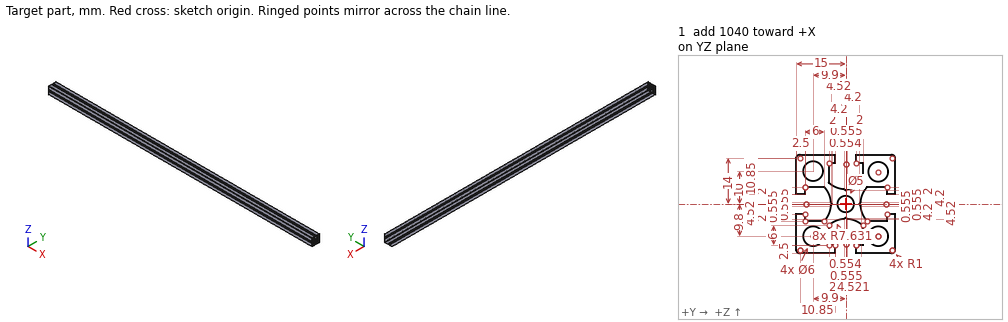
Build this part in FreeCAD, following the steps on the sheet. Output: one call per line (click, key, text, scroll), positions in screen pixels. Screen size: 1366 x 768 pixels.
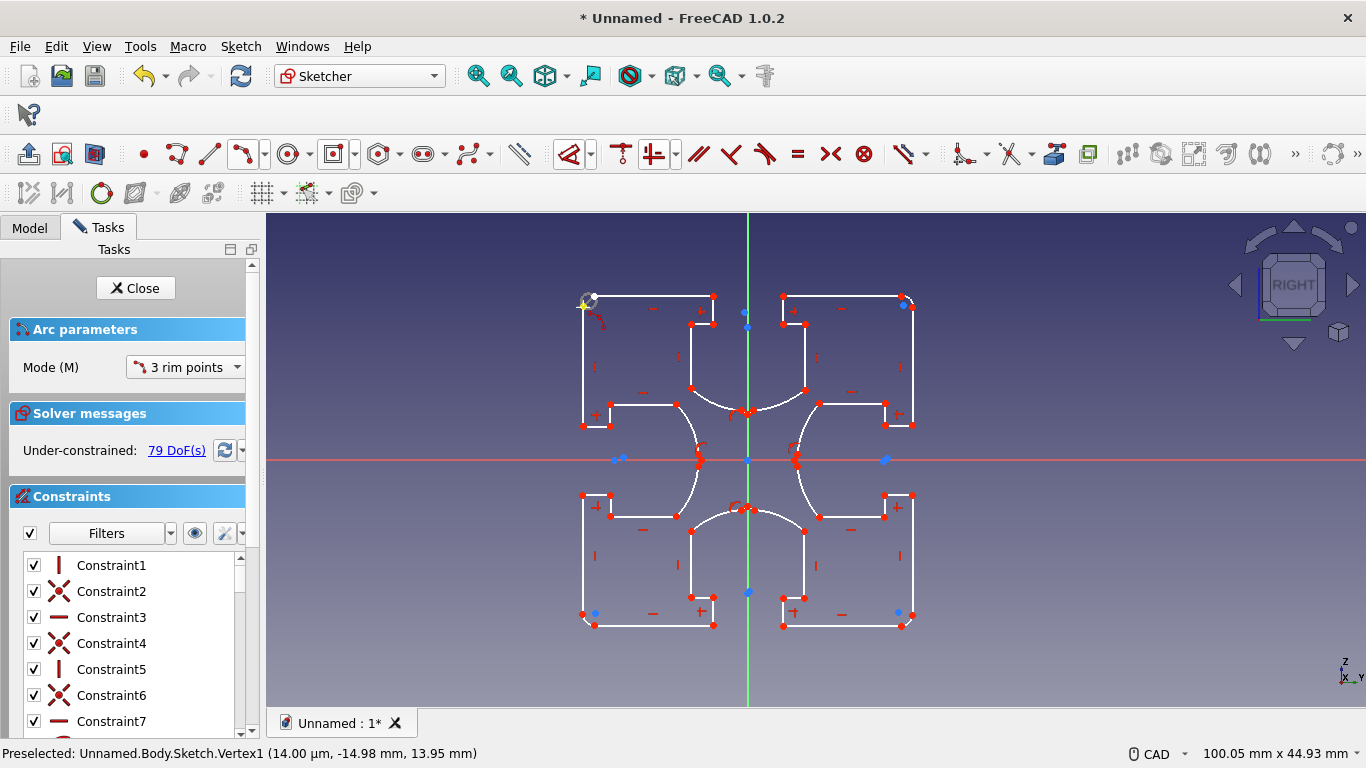
scroll(586, 298, up, 8)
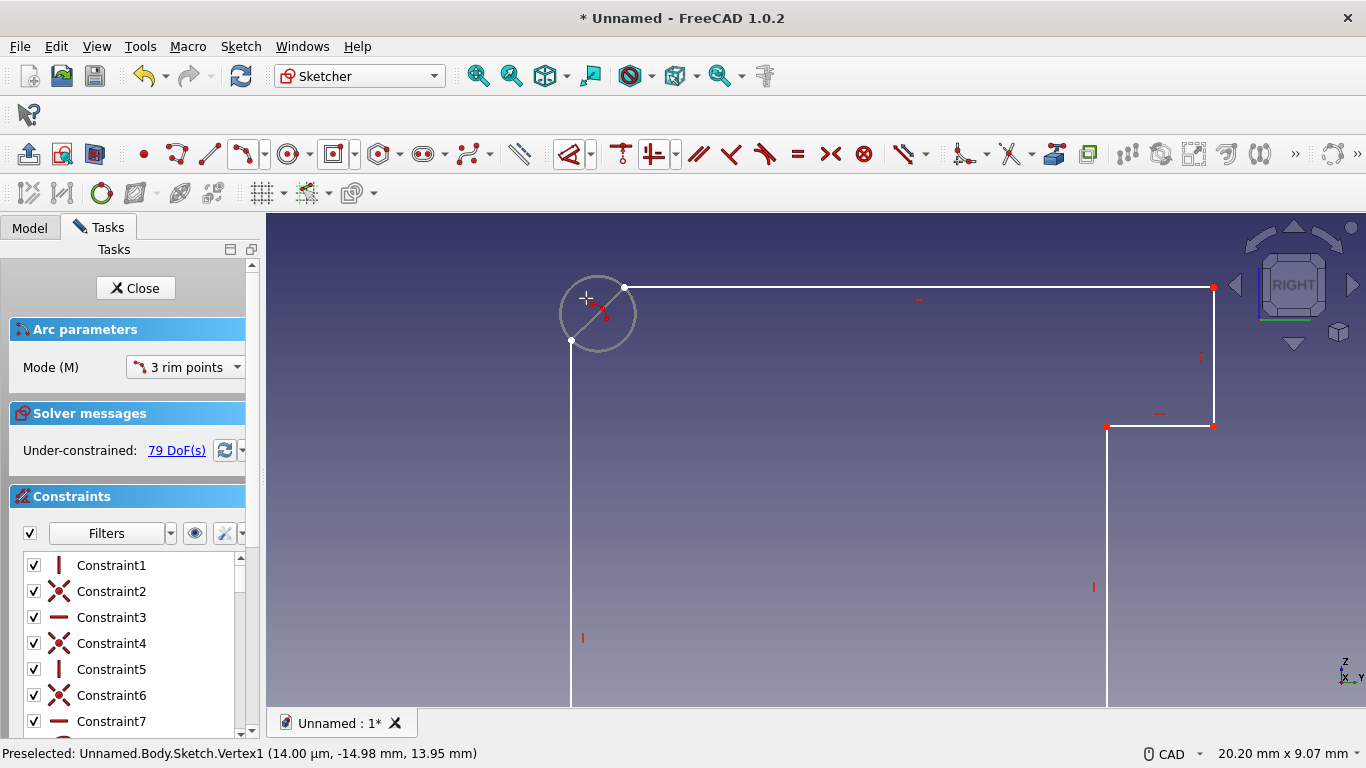
click(586, 299)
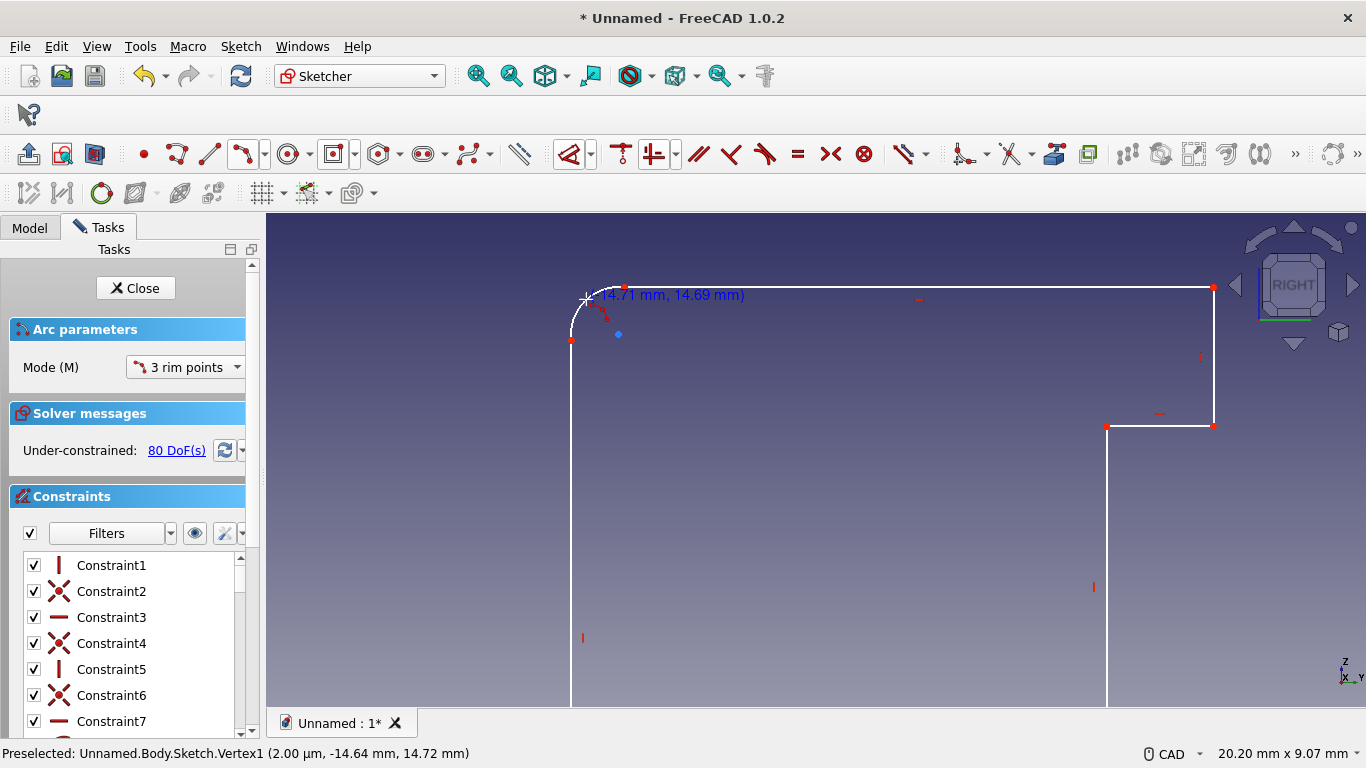
key(g)
key(c)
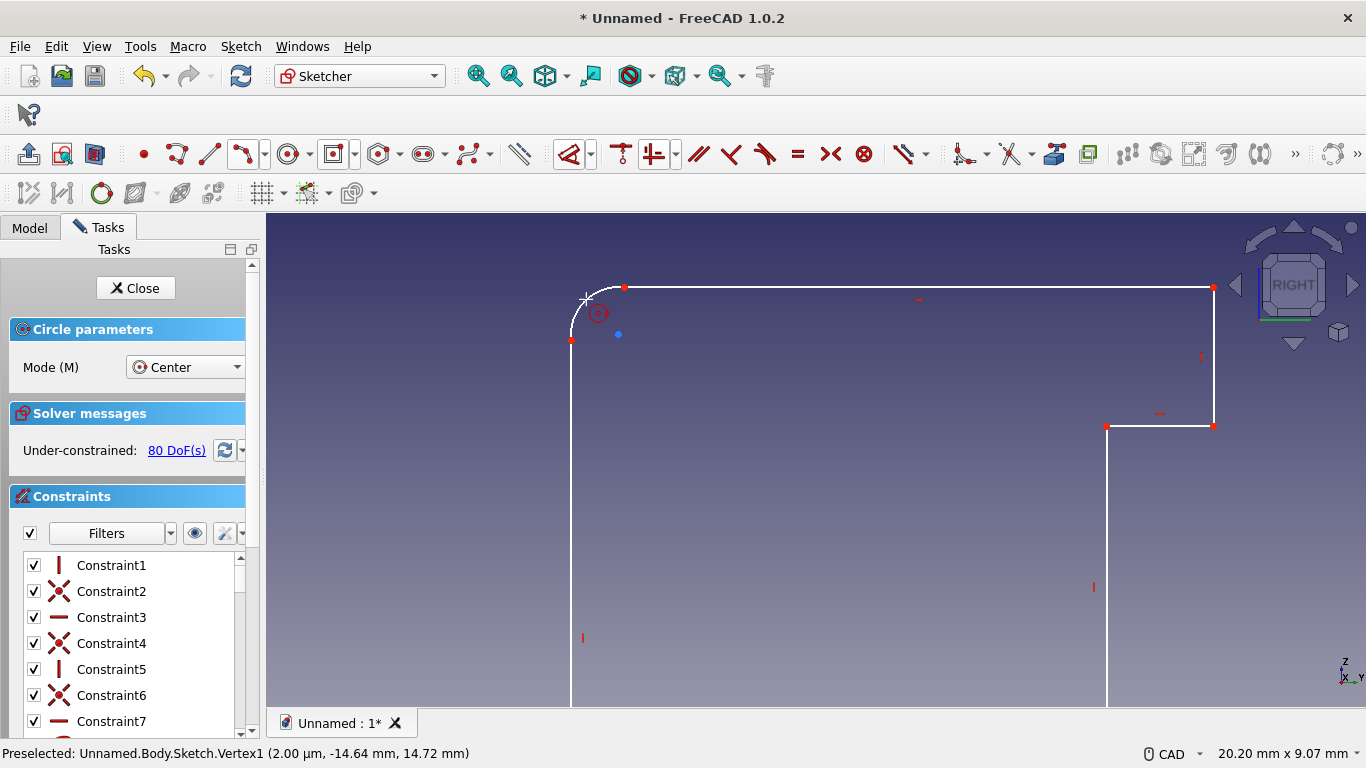
scroll(586, 298, down, 8)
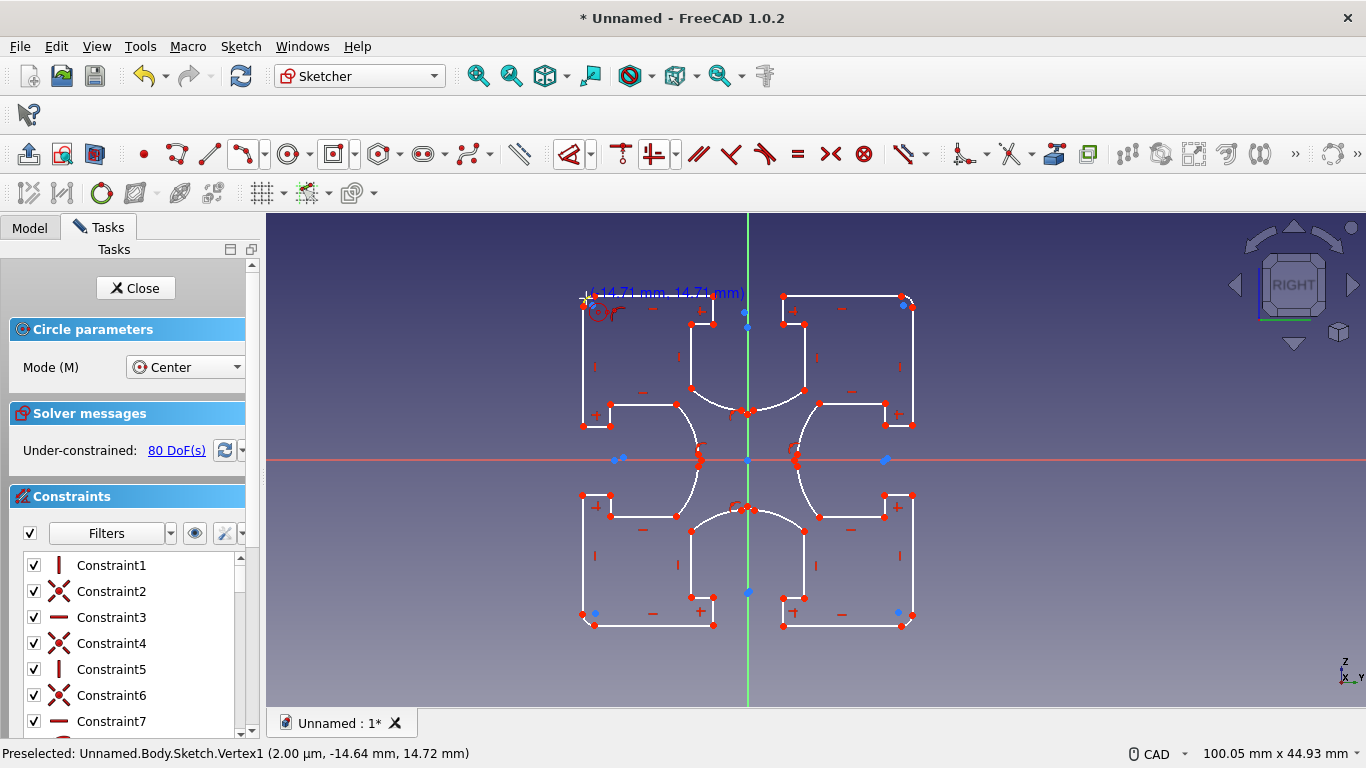
click(639, 350)
click(662, 327)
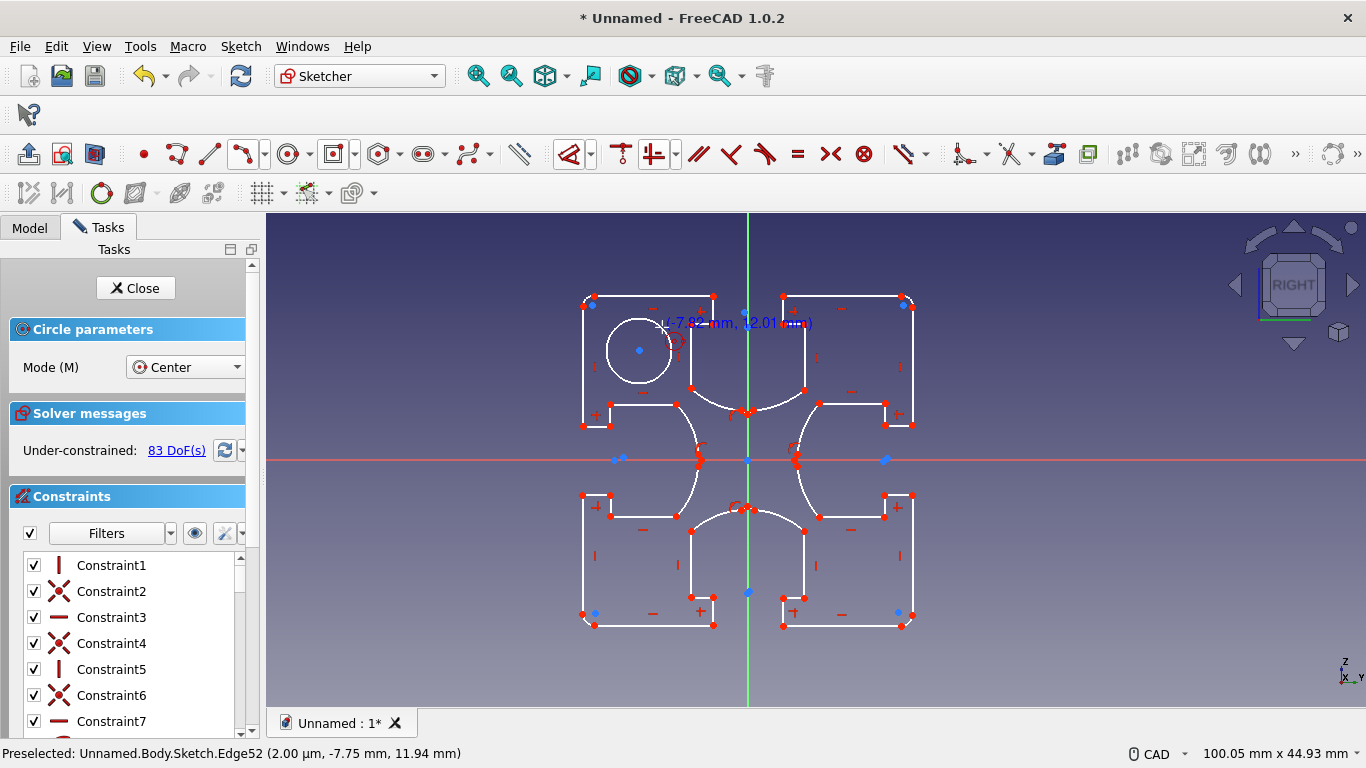
click(639, 568)
click(662, 544)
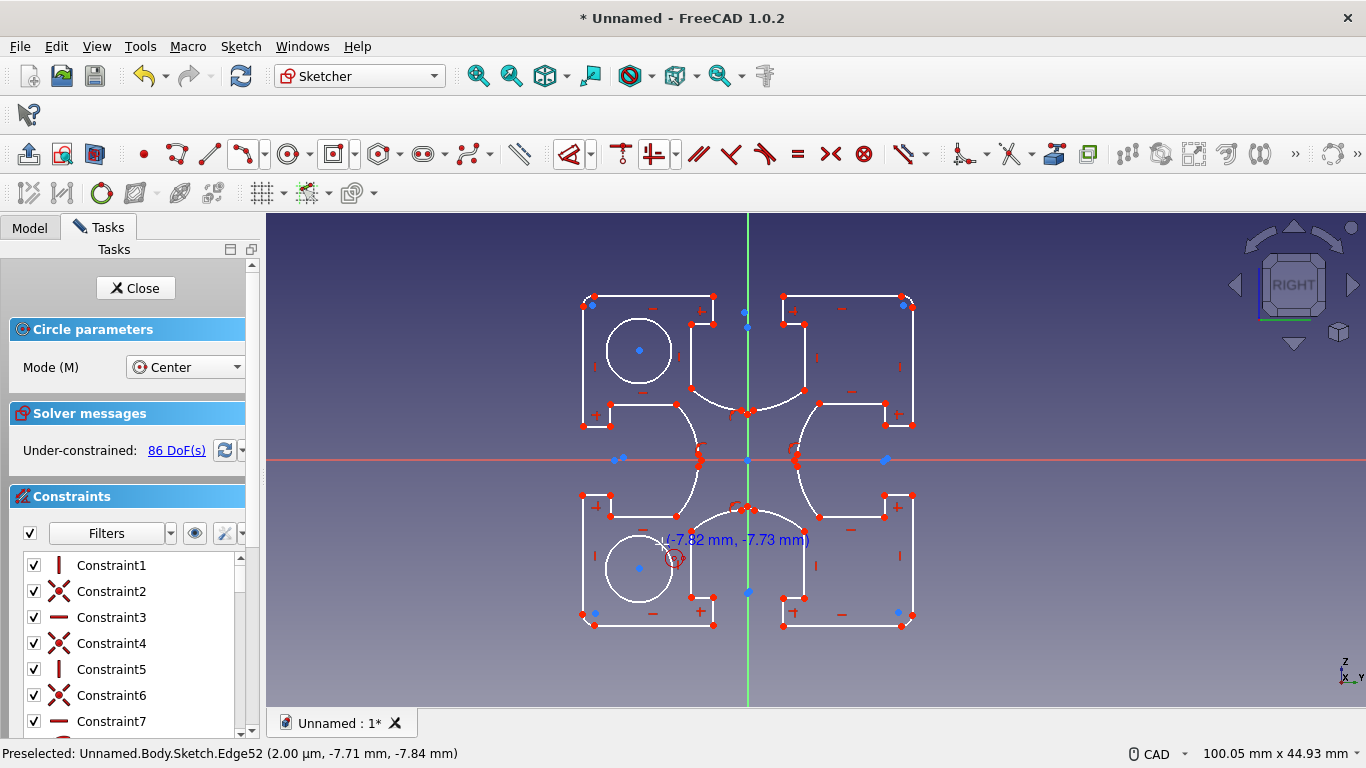
click(857, 352)
click(880, 329)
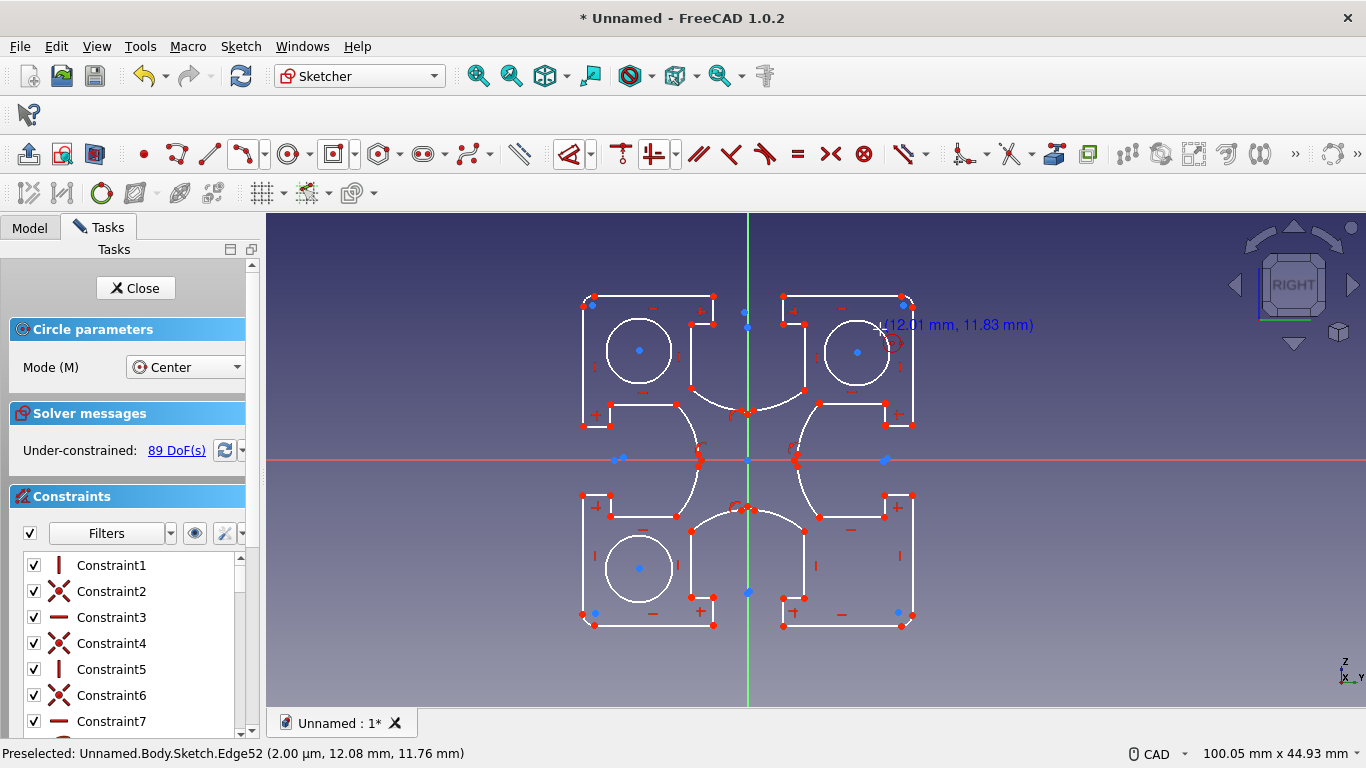
click(748, 460)
click(767, 441)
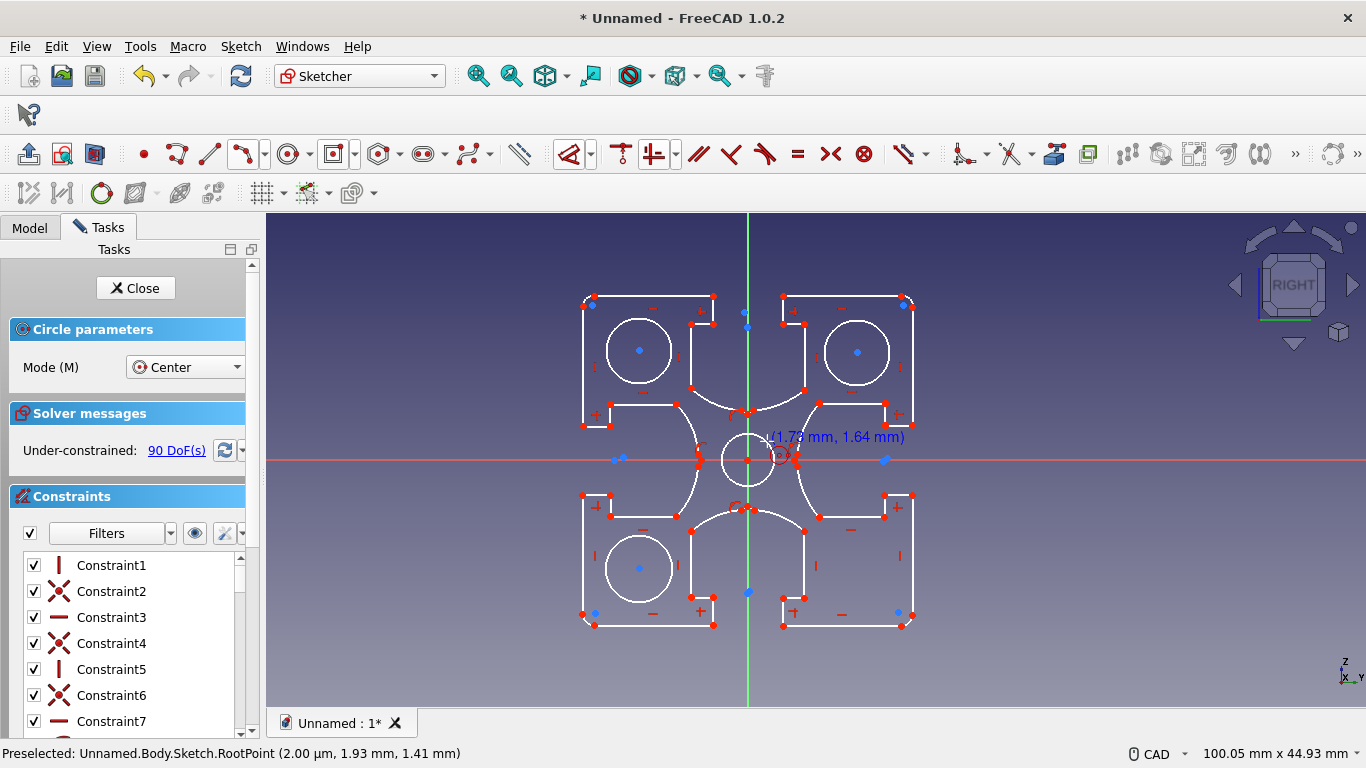
click(857, 568)
click(880, 544)
key(Escape)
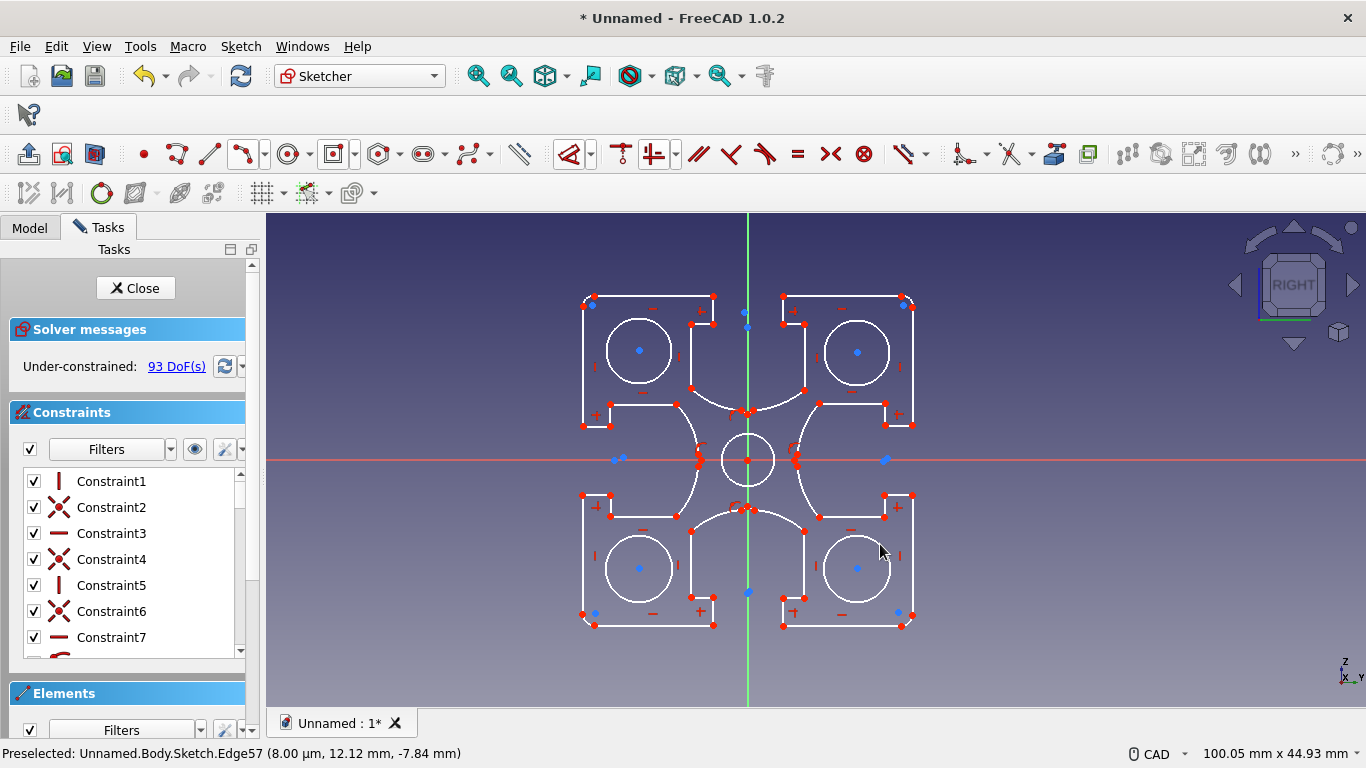
click(583, 343)